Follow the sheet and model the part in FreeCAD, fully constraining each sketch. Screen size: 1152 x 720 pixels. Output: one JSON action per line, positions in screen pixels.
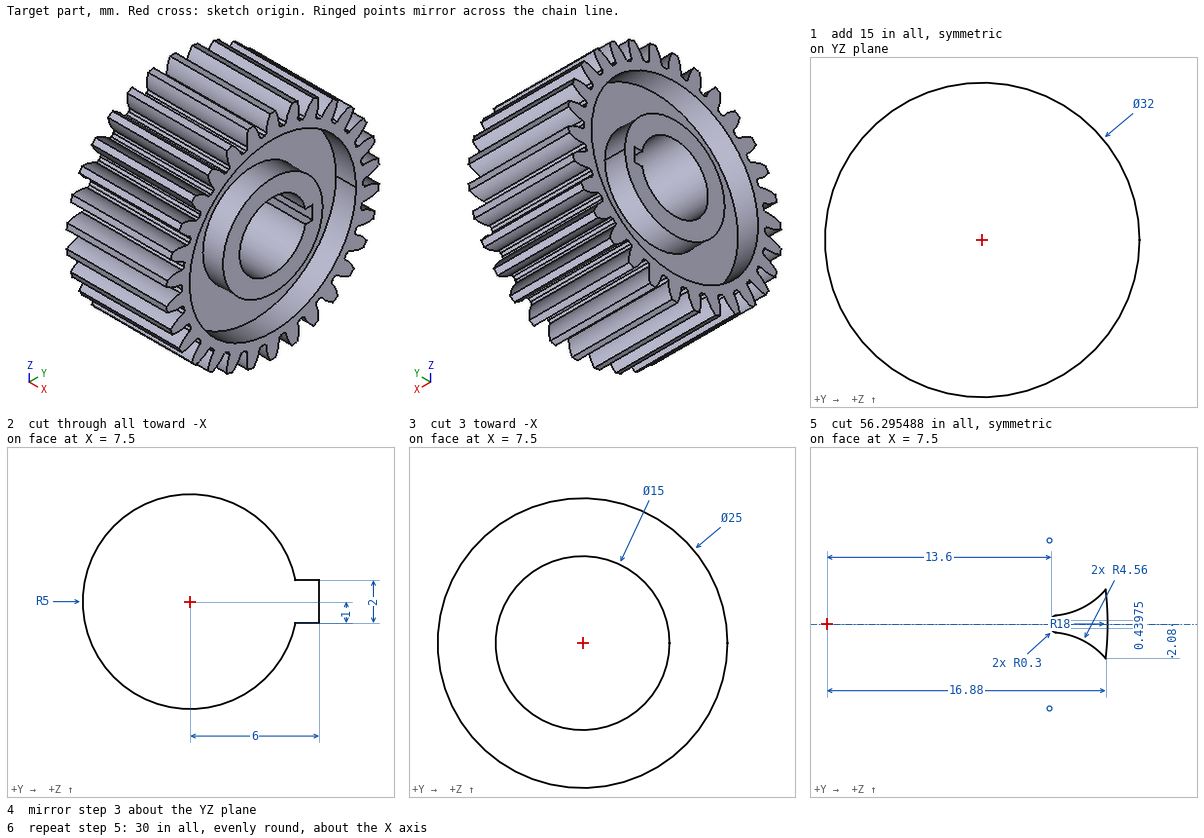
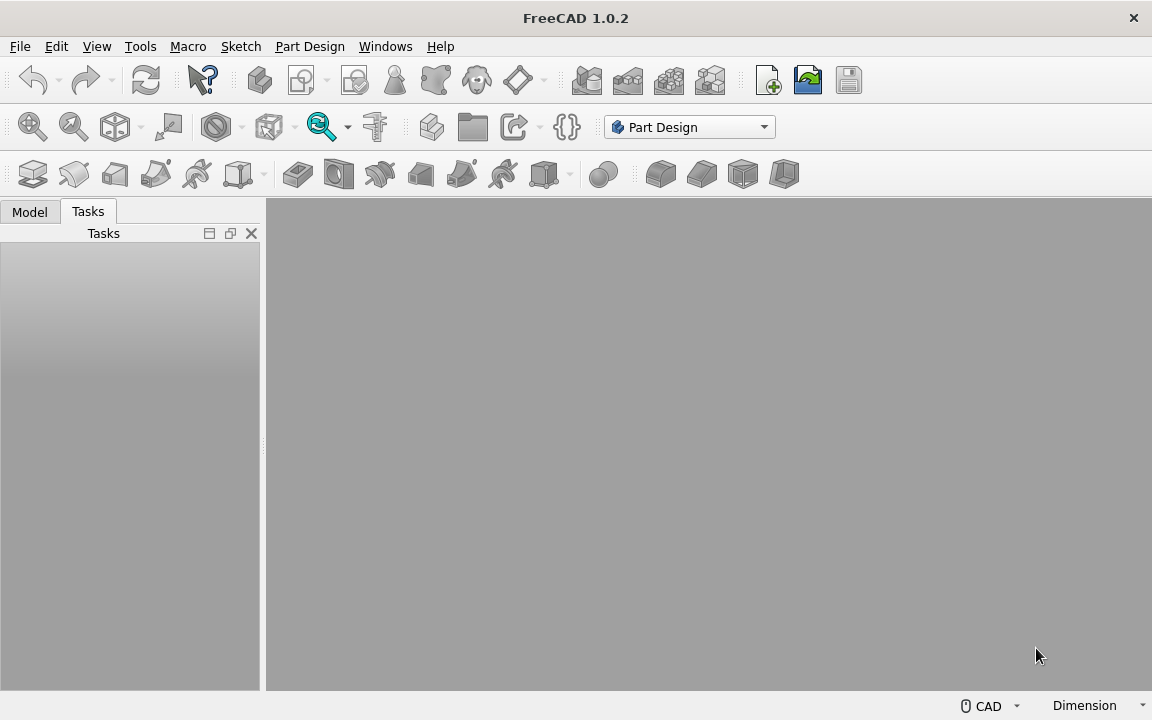
{"action": "left_click", "coordinate": [767, 80]}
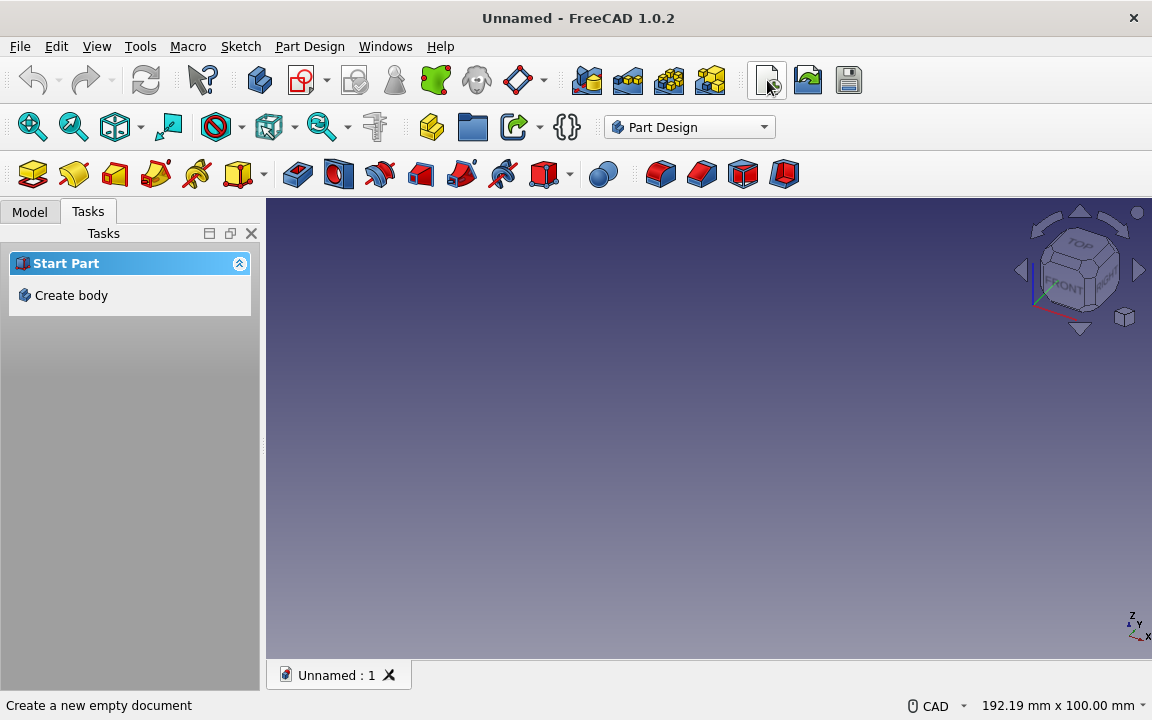
{"action": "left_click", "coordinate": [300, 80]}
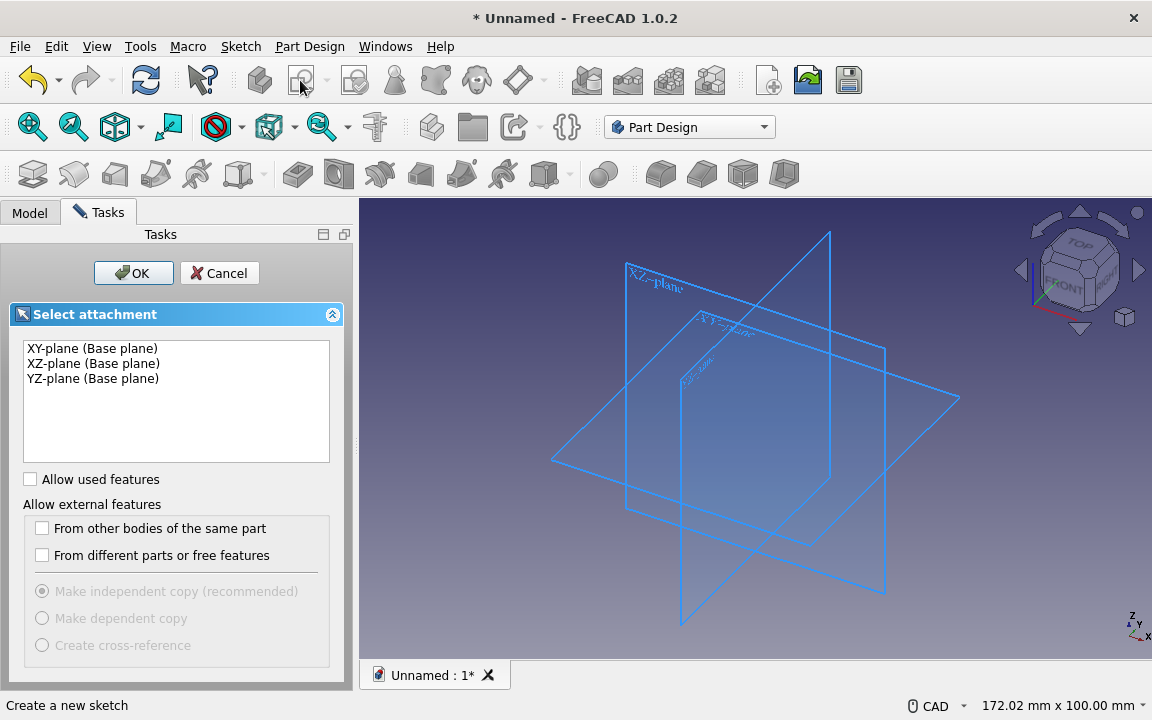
{"action": "left_click", "coordinate": [84, 378]}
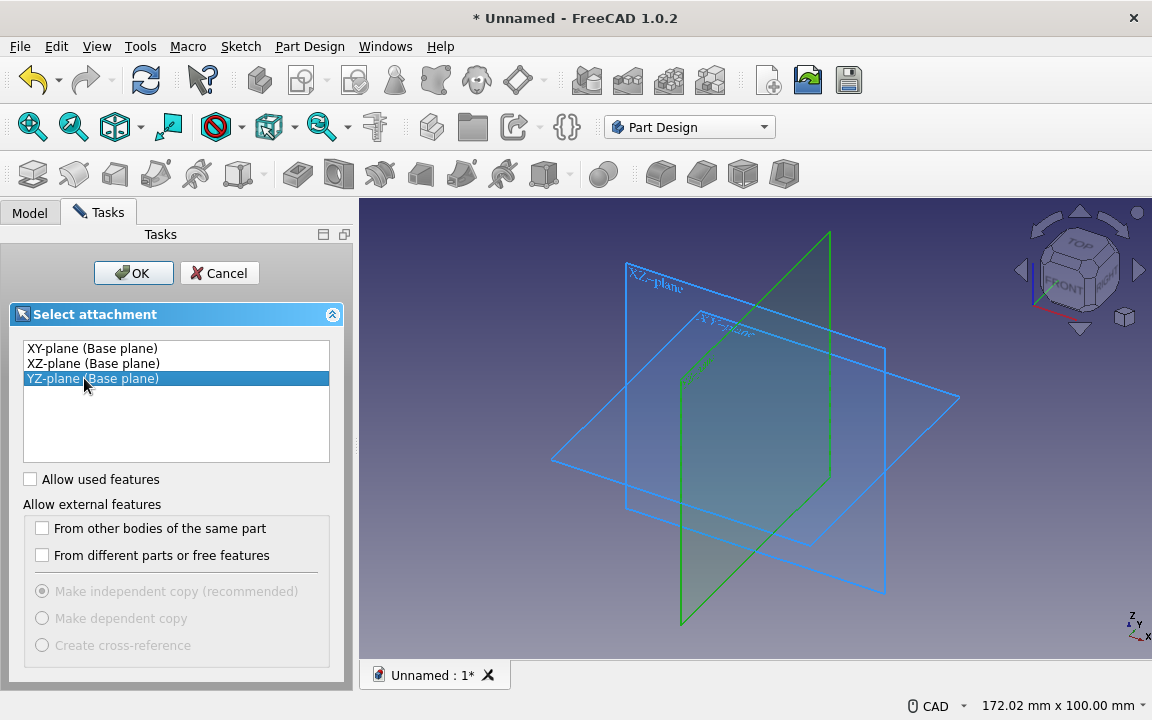
{"action": "left_click", "coordinate": [134, 273]}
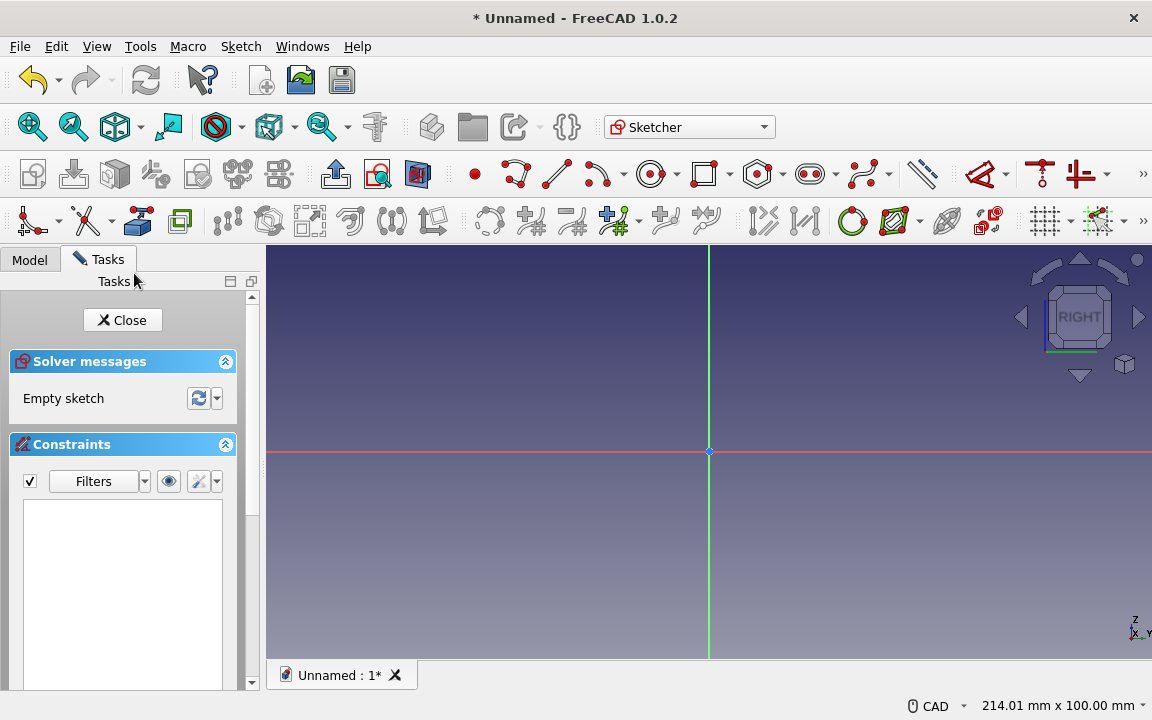
{"action": "scroll", "coordinate": [792, 452], "scroll_direction": "up", "scroll_amount": 3}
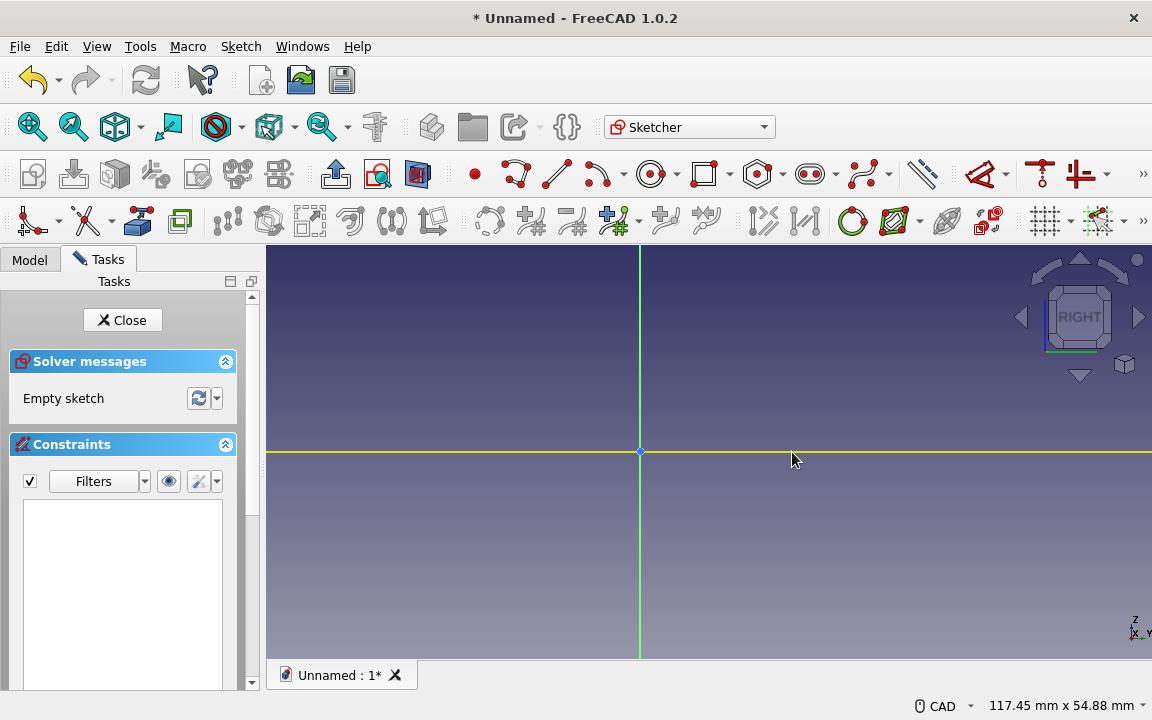
{"action": "key", "text": "g c"}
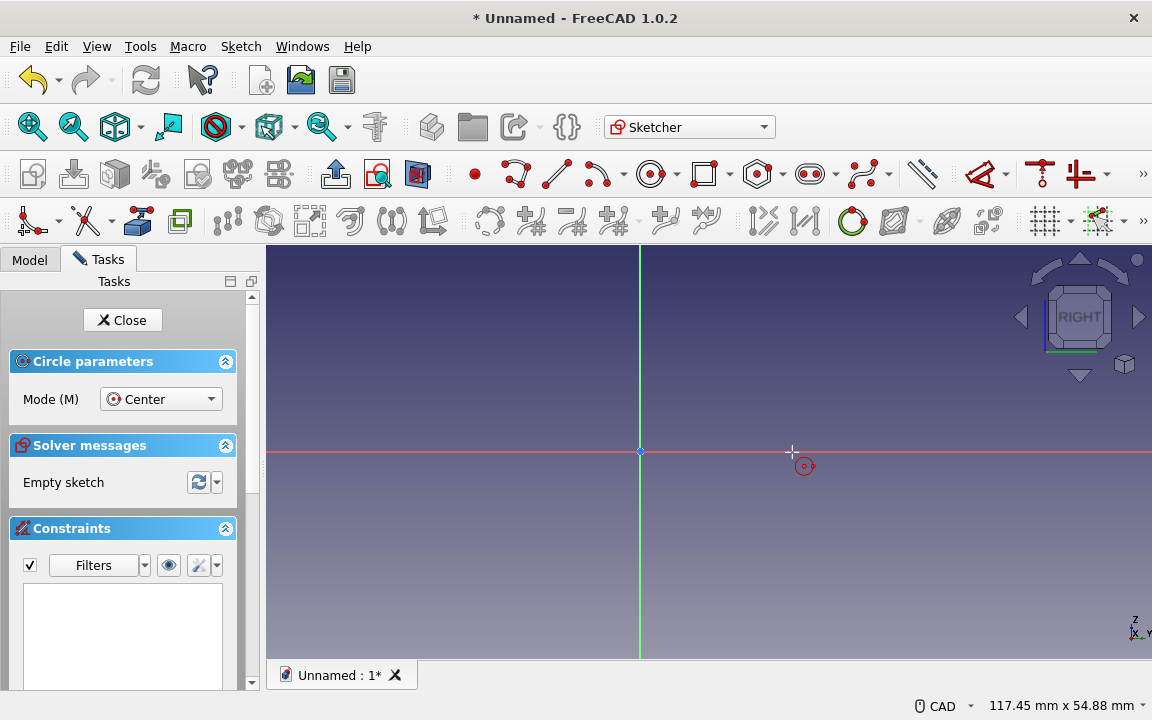
{"action": "left_click", "coordinate": [640, 452]}
{"action": "left_click", "coordinate": [726, 366]}
{"action": "key", "text": "Escape"}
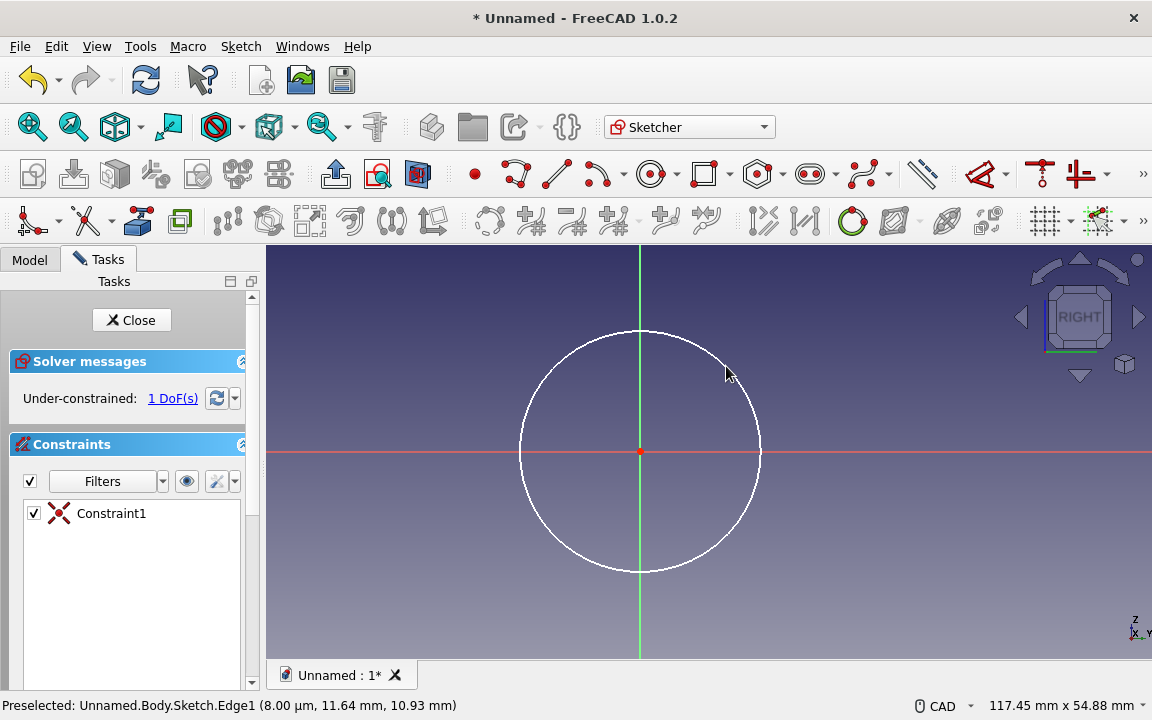
{"action": "left_click", "coordinate": [725, 366]}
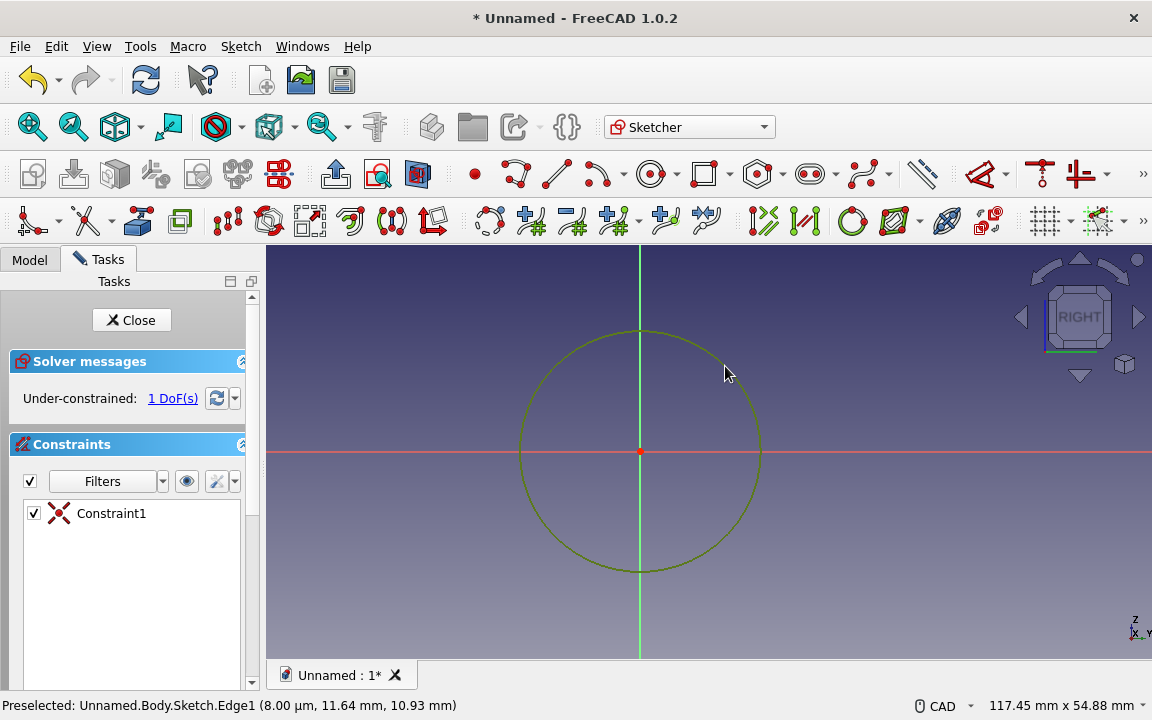
{"action": "key", "text": "k o"}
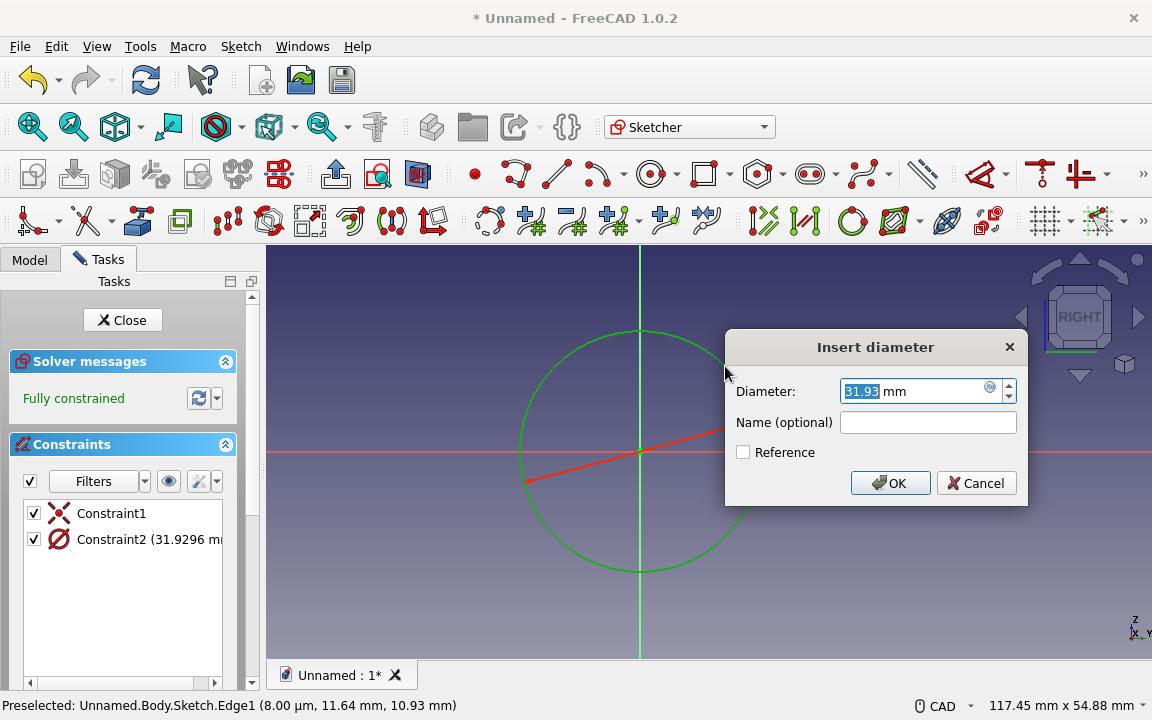
{"action": "type", "text": "32"}
{"action": "key", "text": "Return"}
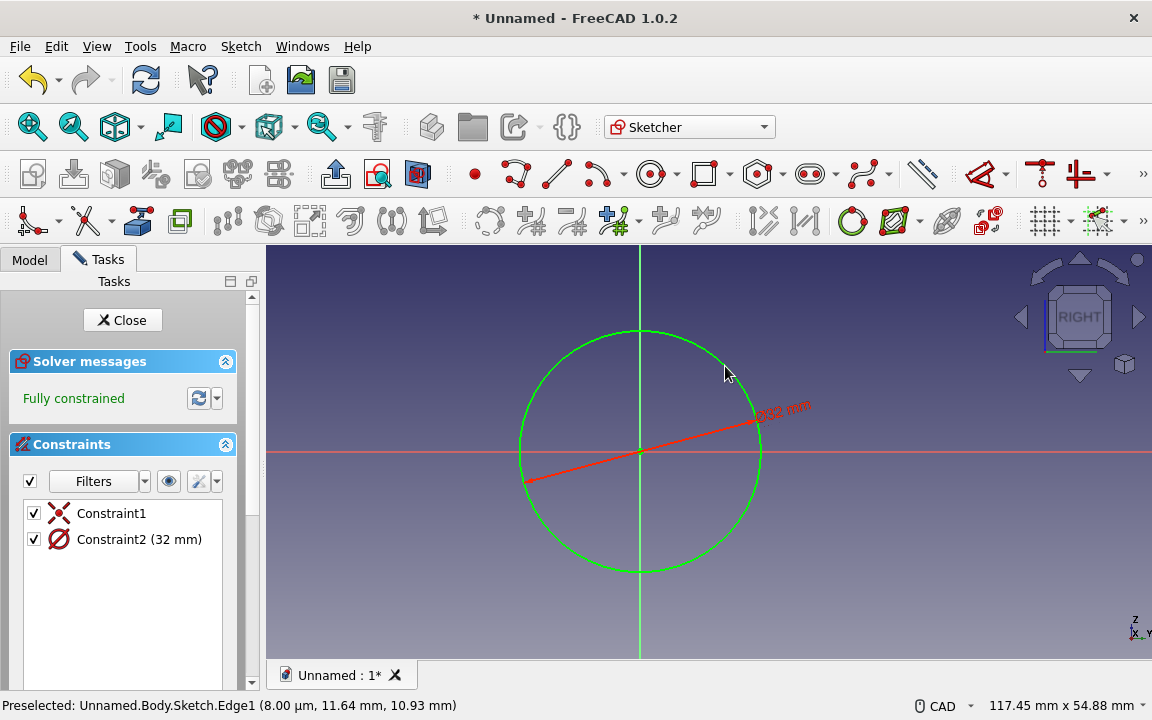
{"action": "left_click", "coordinate": [123, 320]}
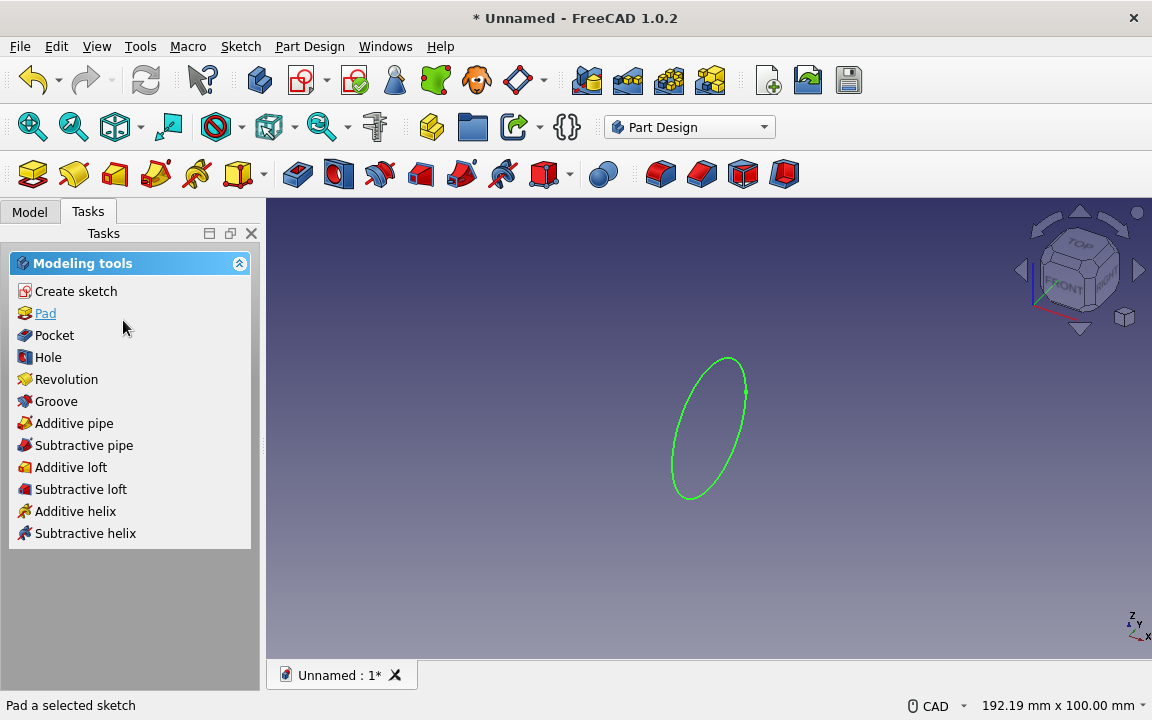
{"action": "left_click", "coordinate": [33, 174]}